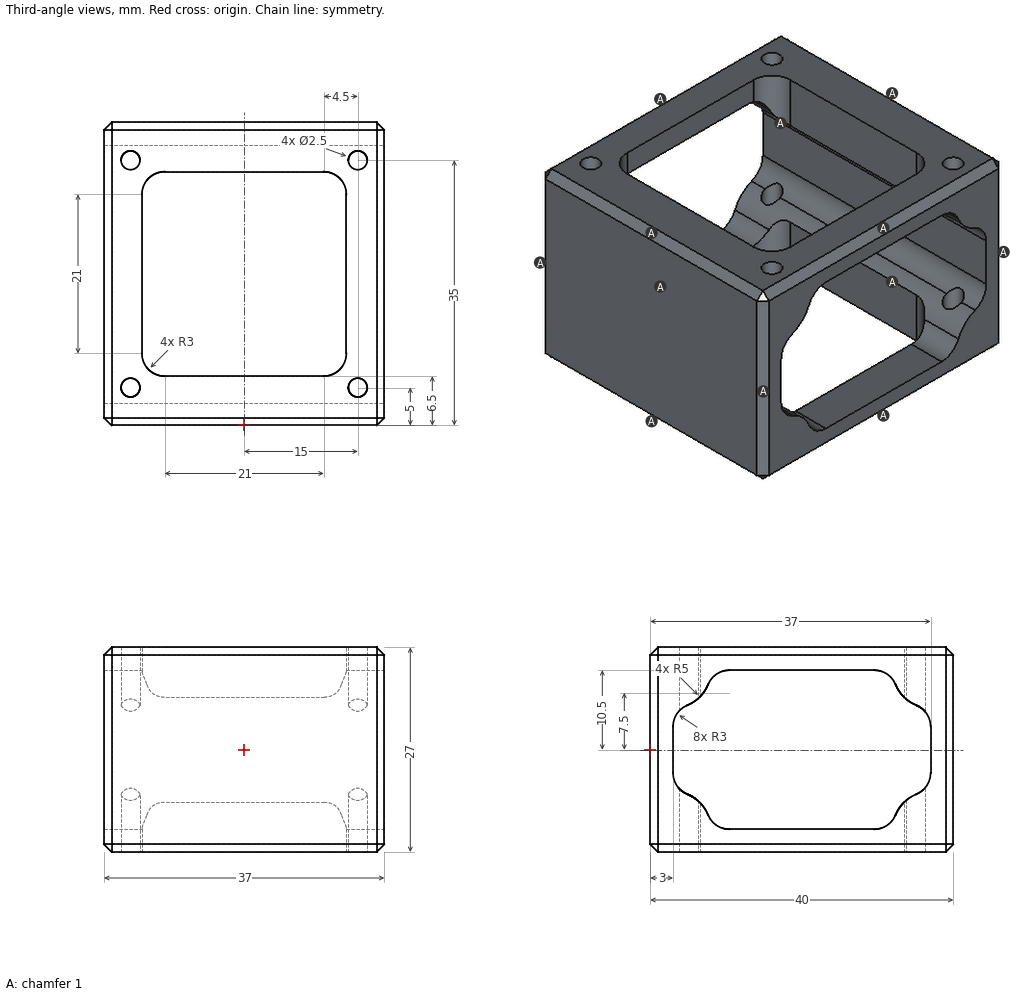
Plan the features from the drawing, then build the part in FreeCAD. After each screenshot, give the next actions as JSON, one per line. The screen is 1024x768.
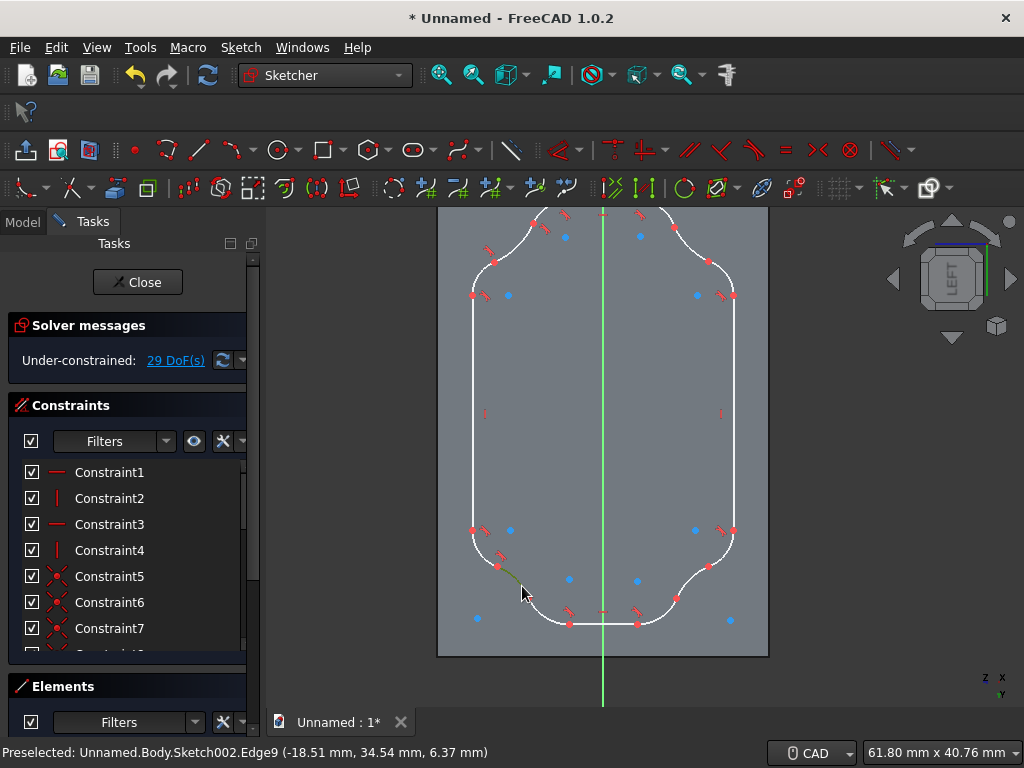
{"action": "left_click", "coordinate": [538, 611]}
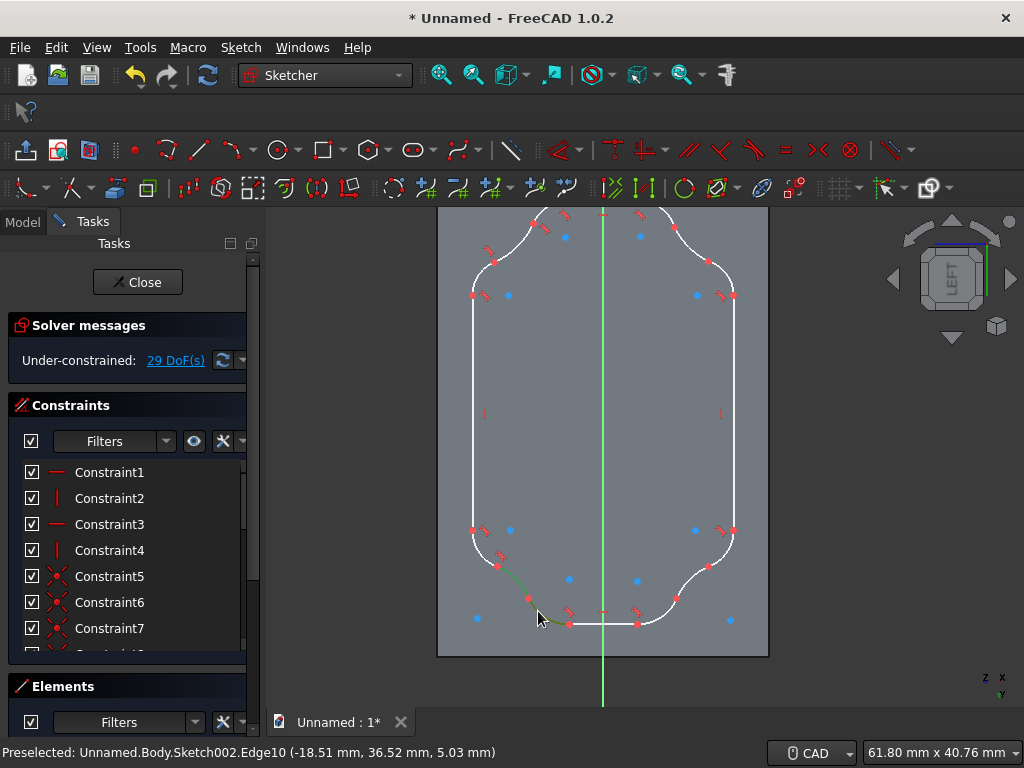
{"action": "key", "text": "t"}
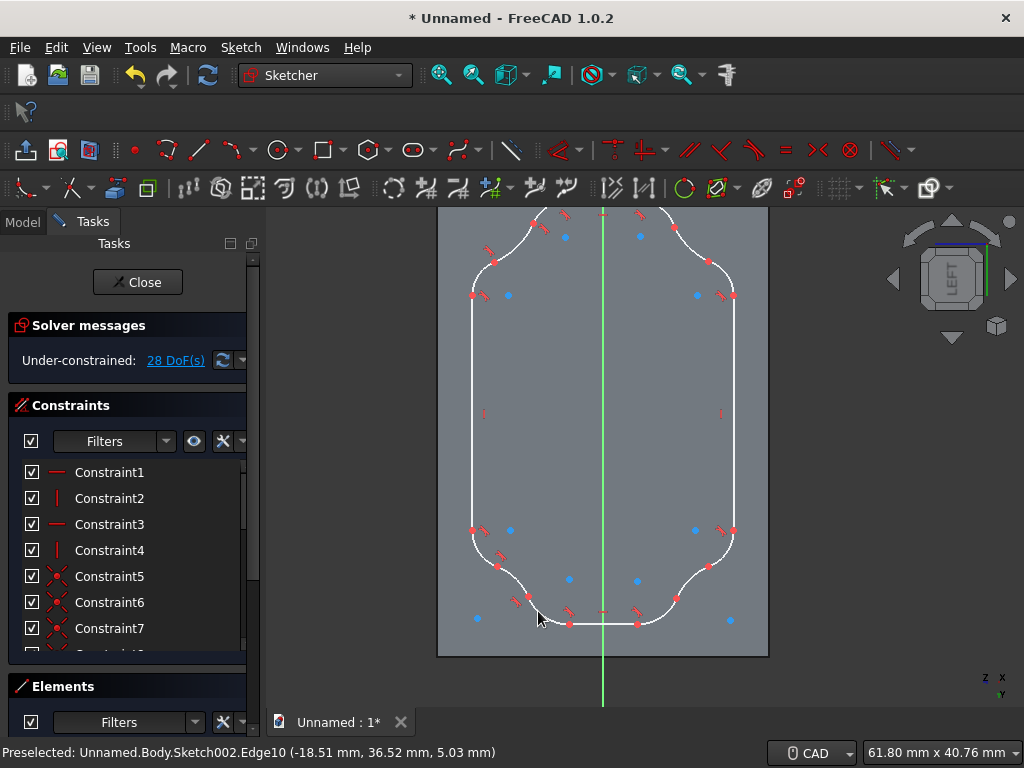
{"action": "left_click", "coordinate": [652, 622]}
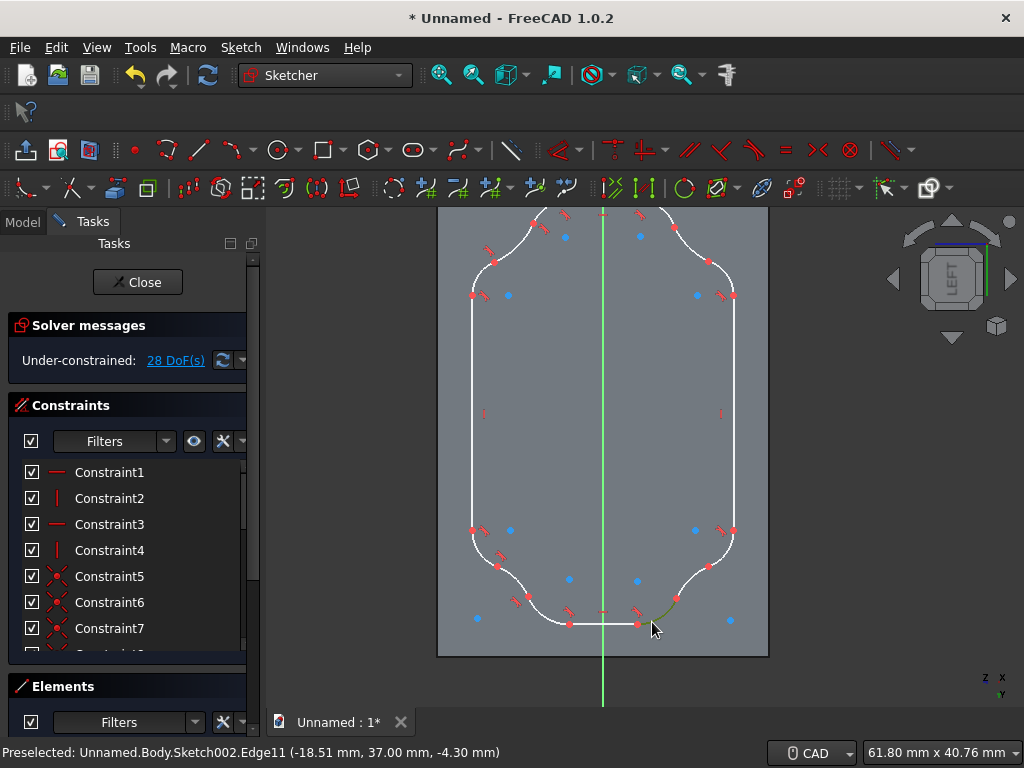
{"action": "left_click", "coordinate": [697, 573]}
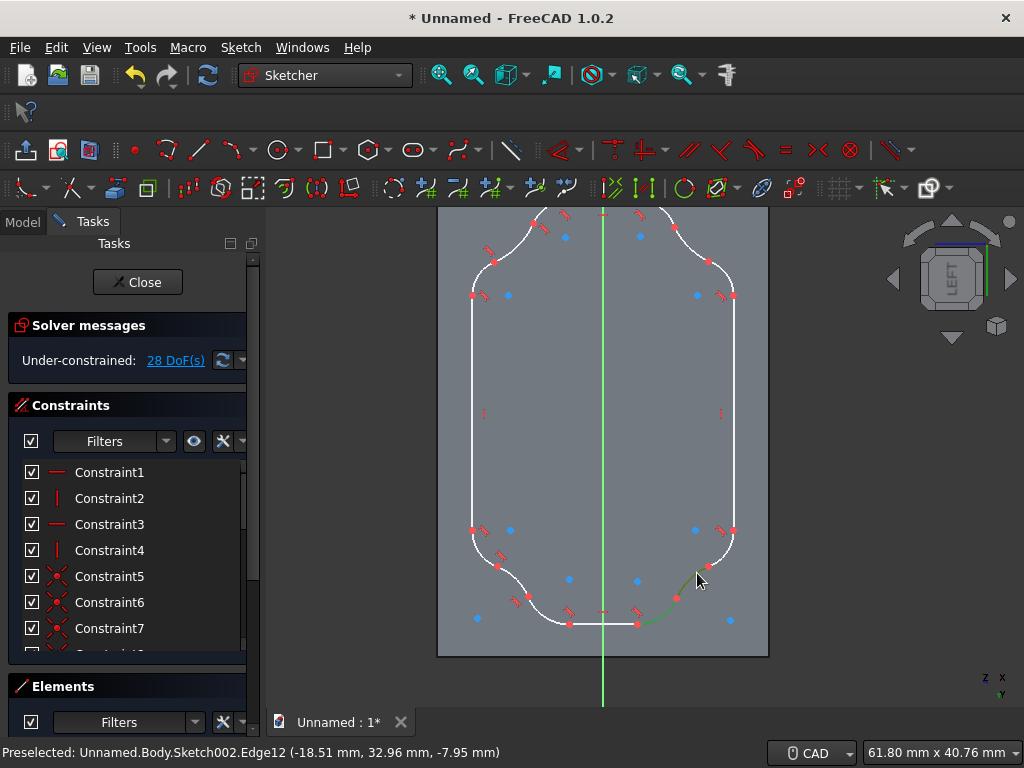
{"action": "key", "text": "t"}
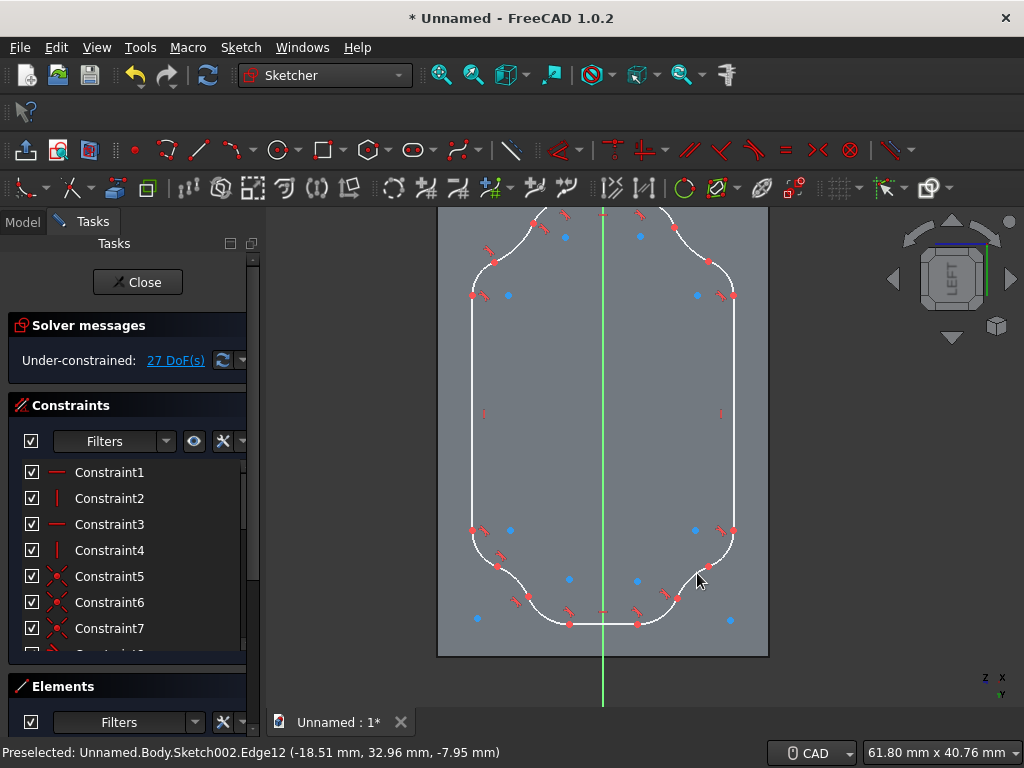
{"action": "left_click", "coordinate": [697, 573]}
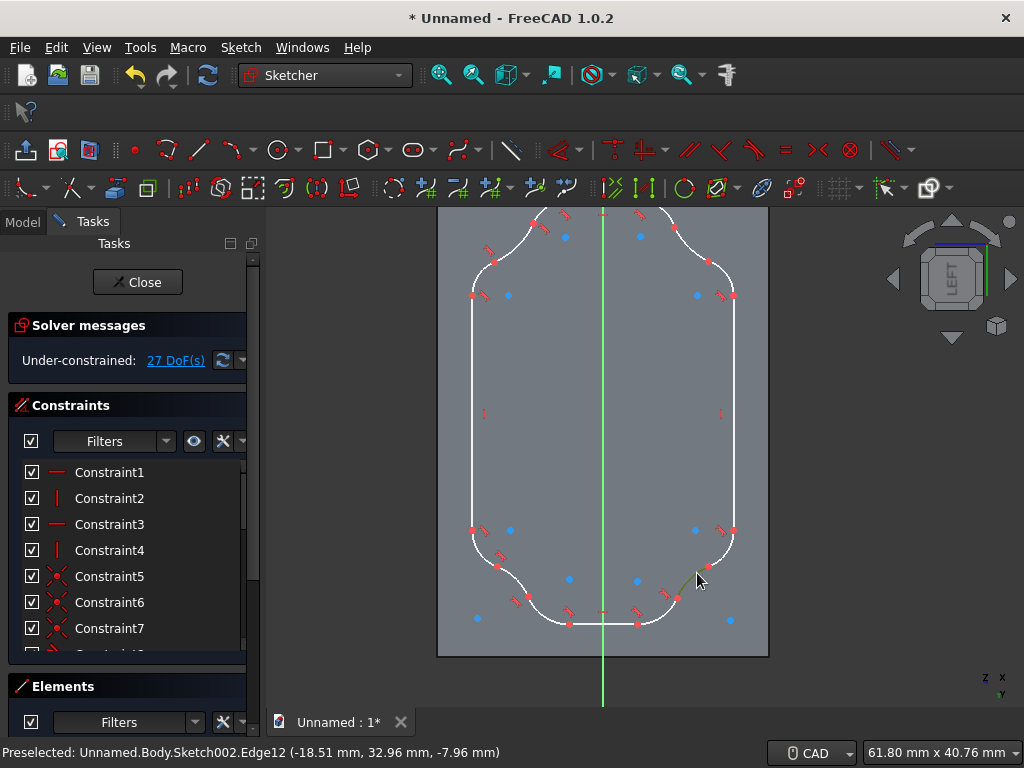
{"action": "left_click", "coordinate": [721, 559]}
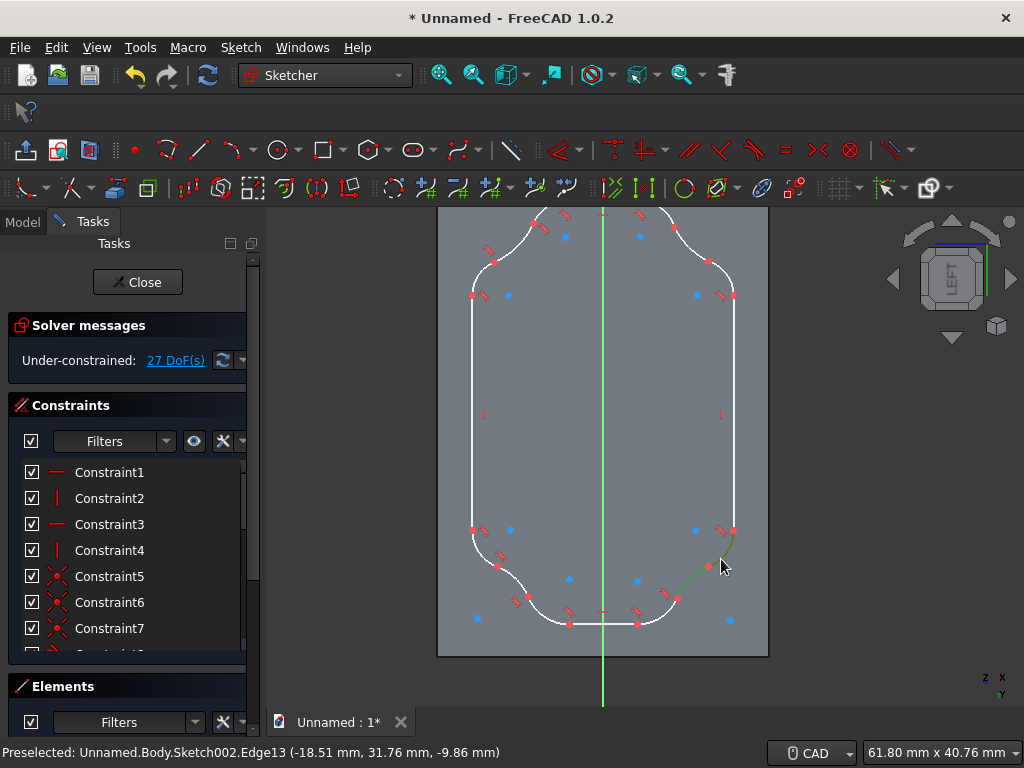
{"action": "left_click", "coordinate": [754, 150]}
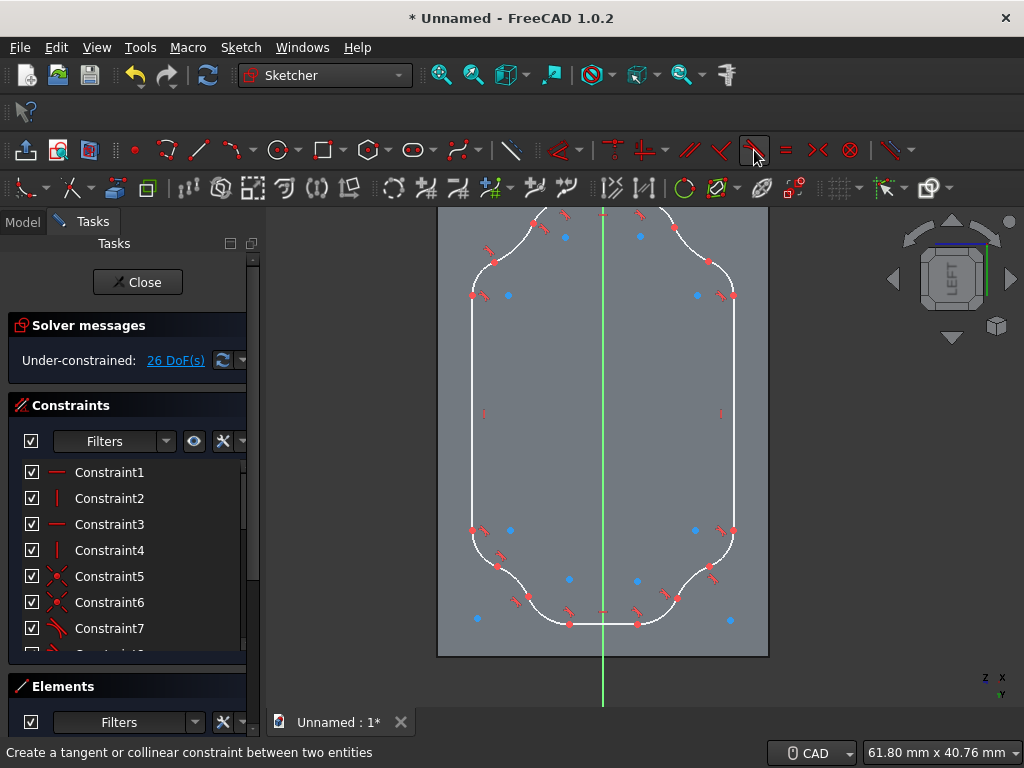
{"action": "left_click", "coordinate": [731, 282]}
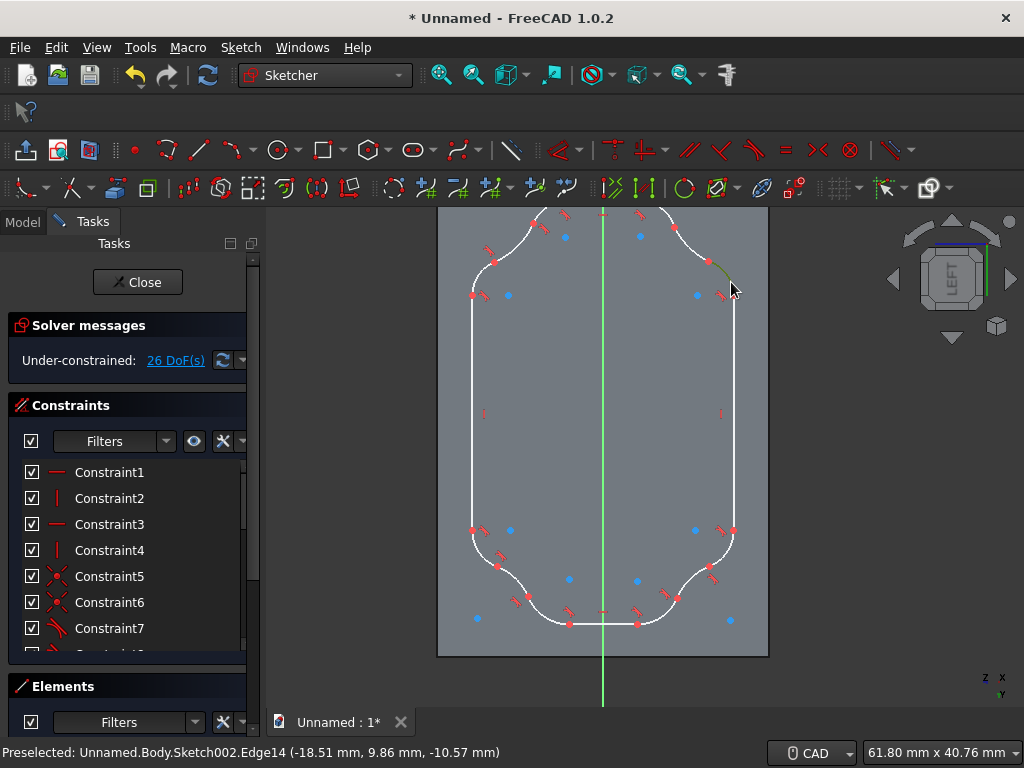
{"action": "left_click", "coordinate": [682, 240]}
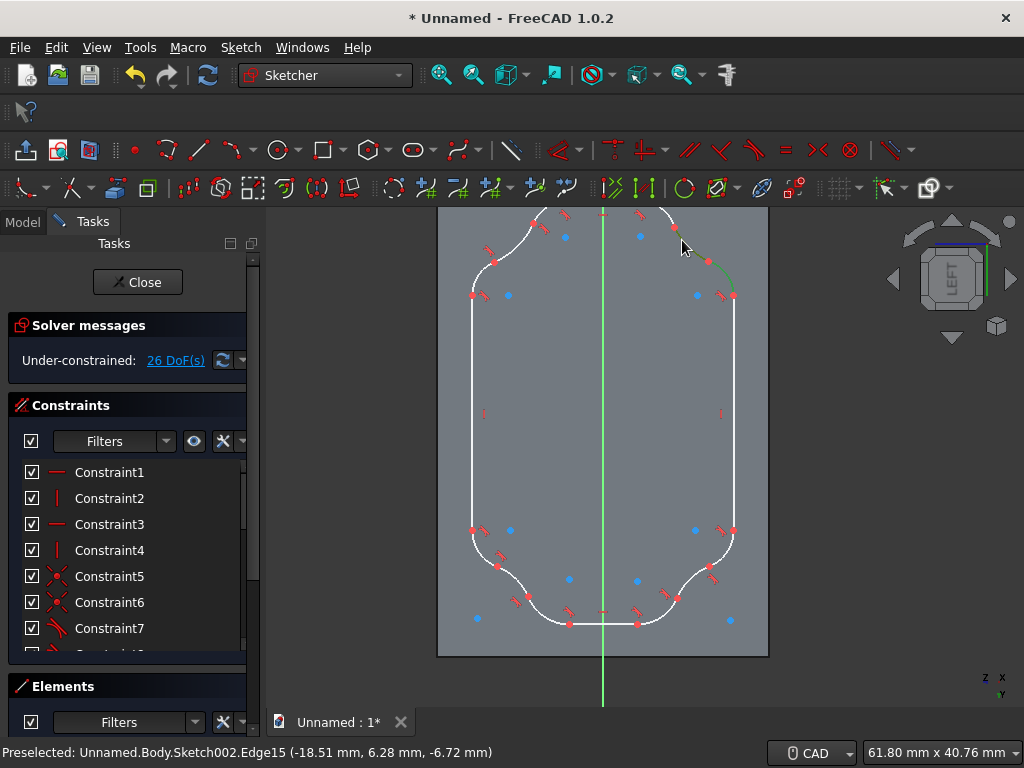
{"action": "key", "text": "t"}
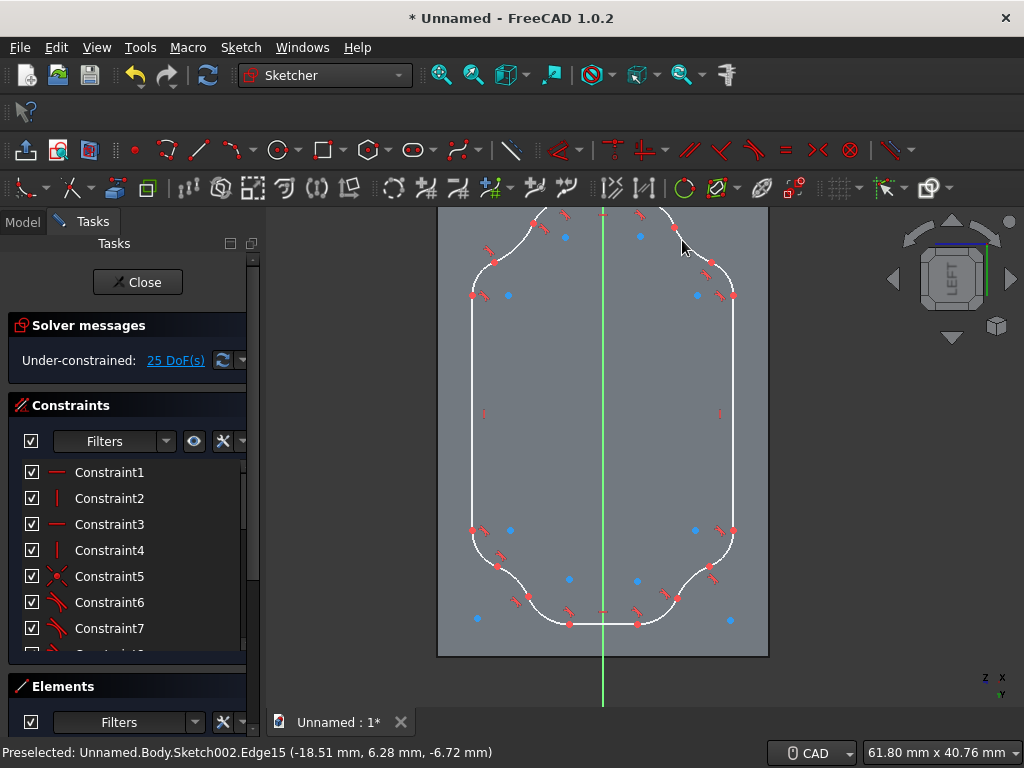
{"action": "left_click", "coordinate": [683, 240]}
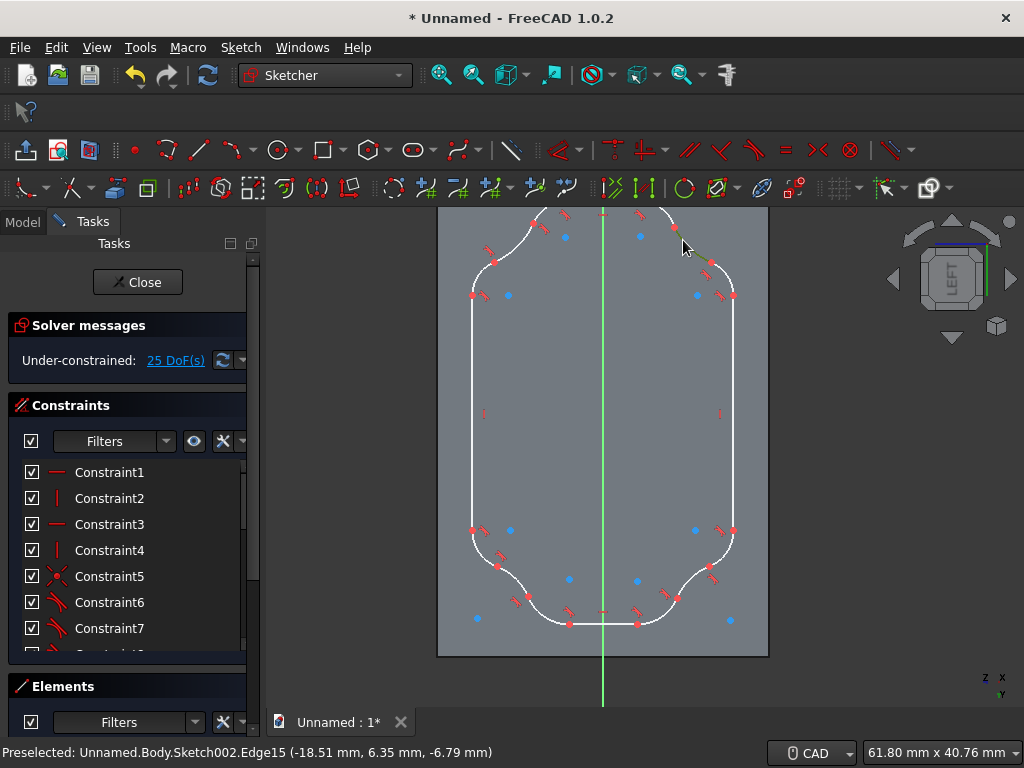
{"action": "scroll", "coordinate": [523, 586], "scroll_direction": "down", "scroll_amount": 2}